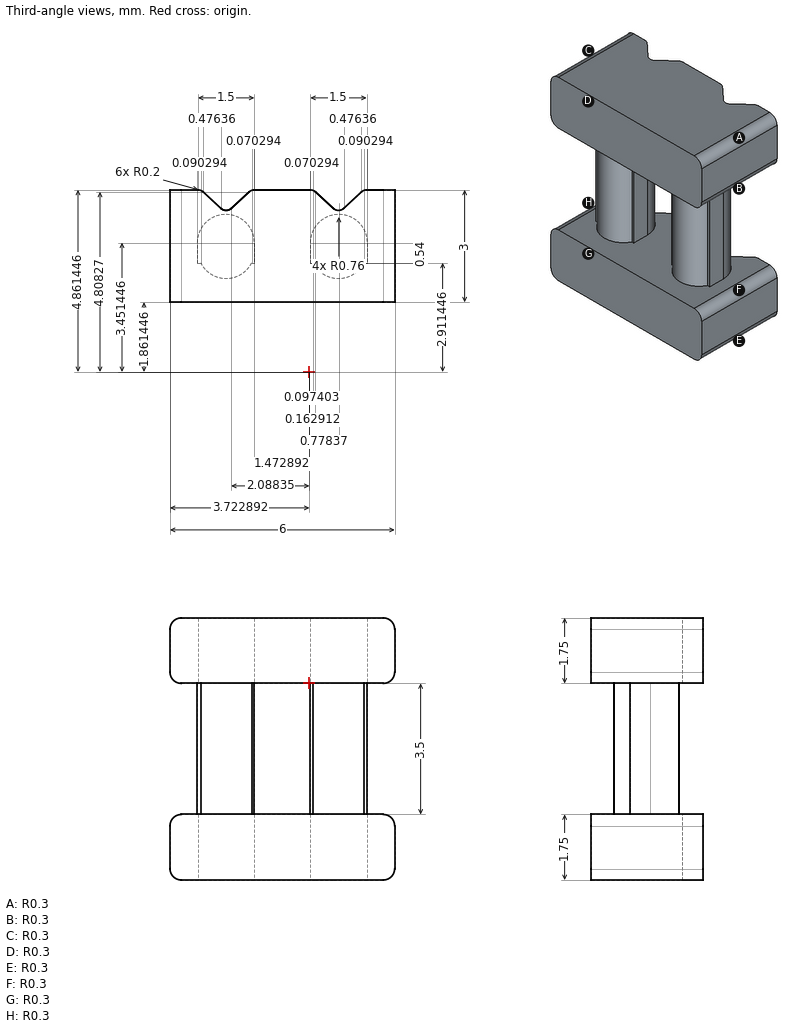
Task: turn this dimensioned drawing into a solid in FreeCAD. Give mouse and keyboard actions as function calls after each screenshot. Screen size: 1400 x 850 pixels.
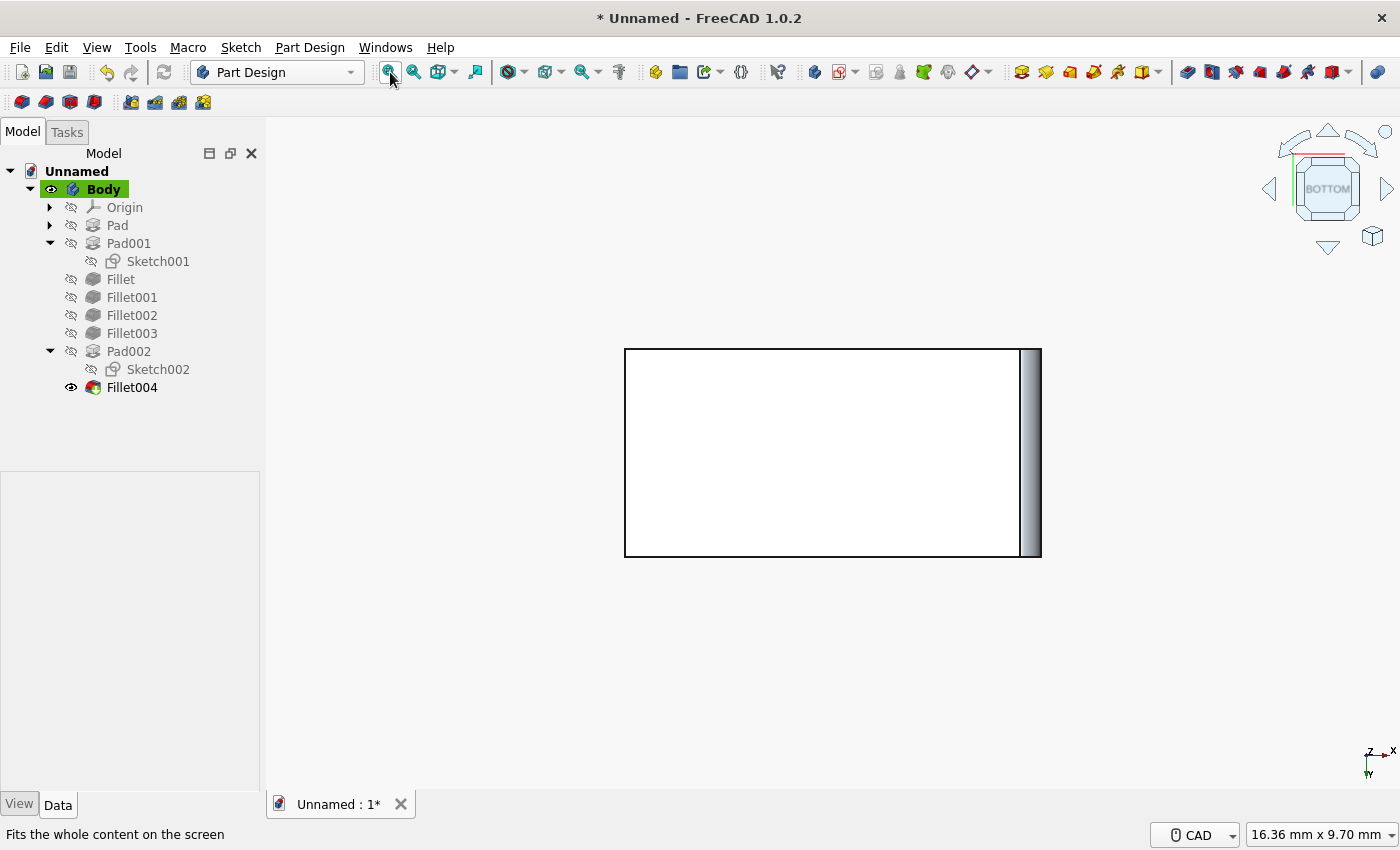
key(0)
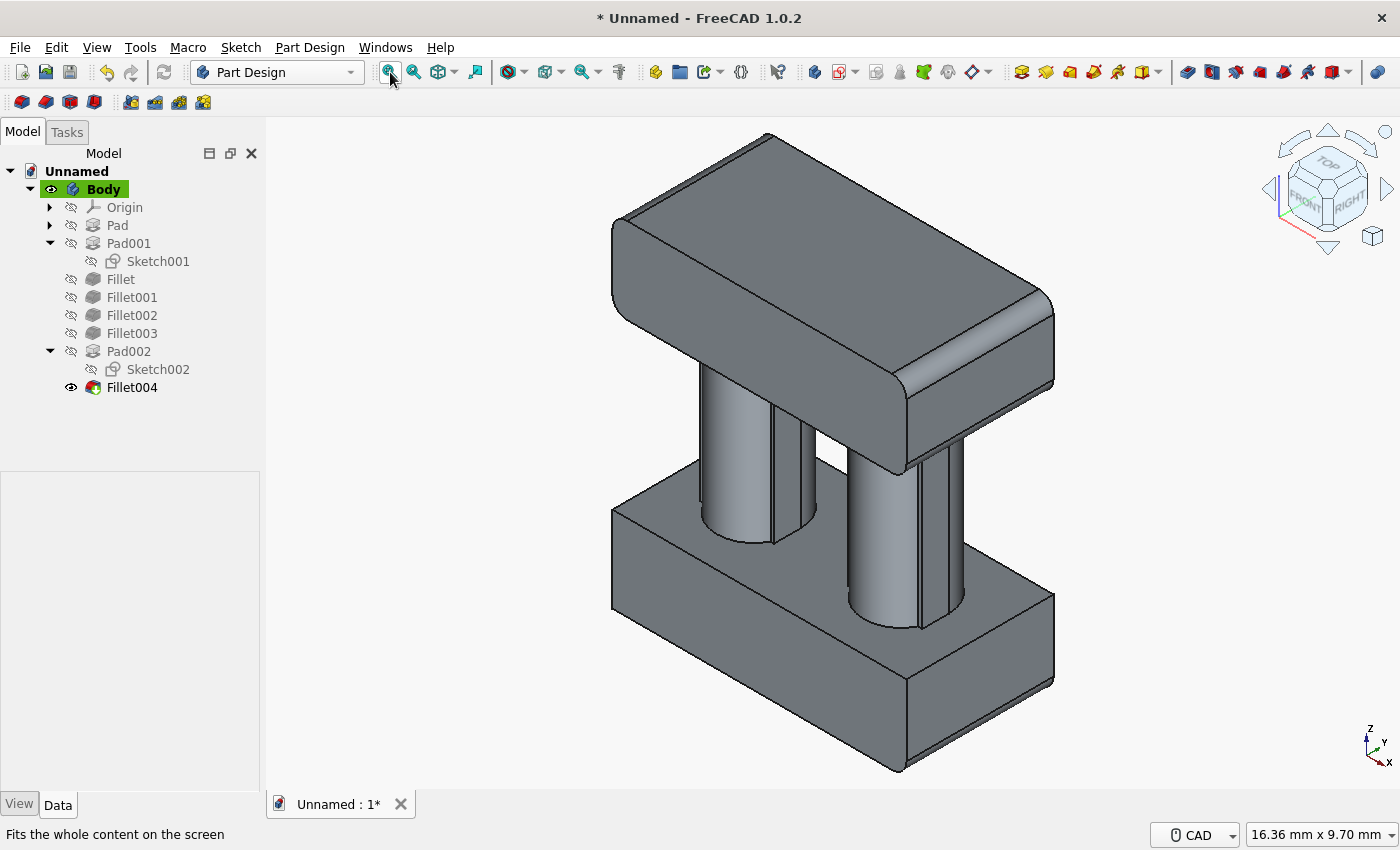
click(980, 636)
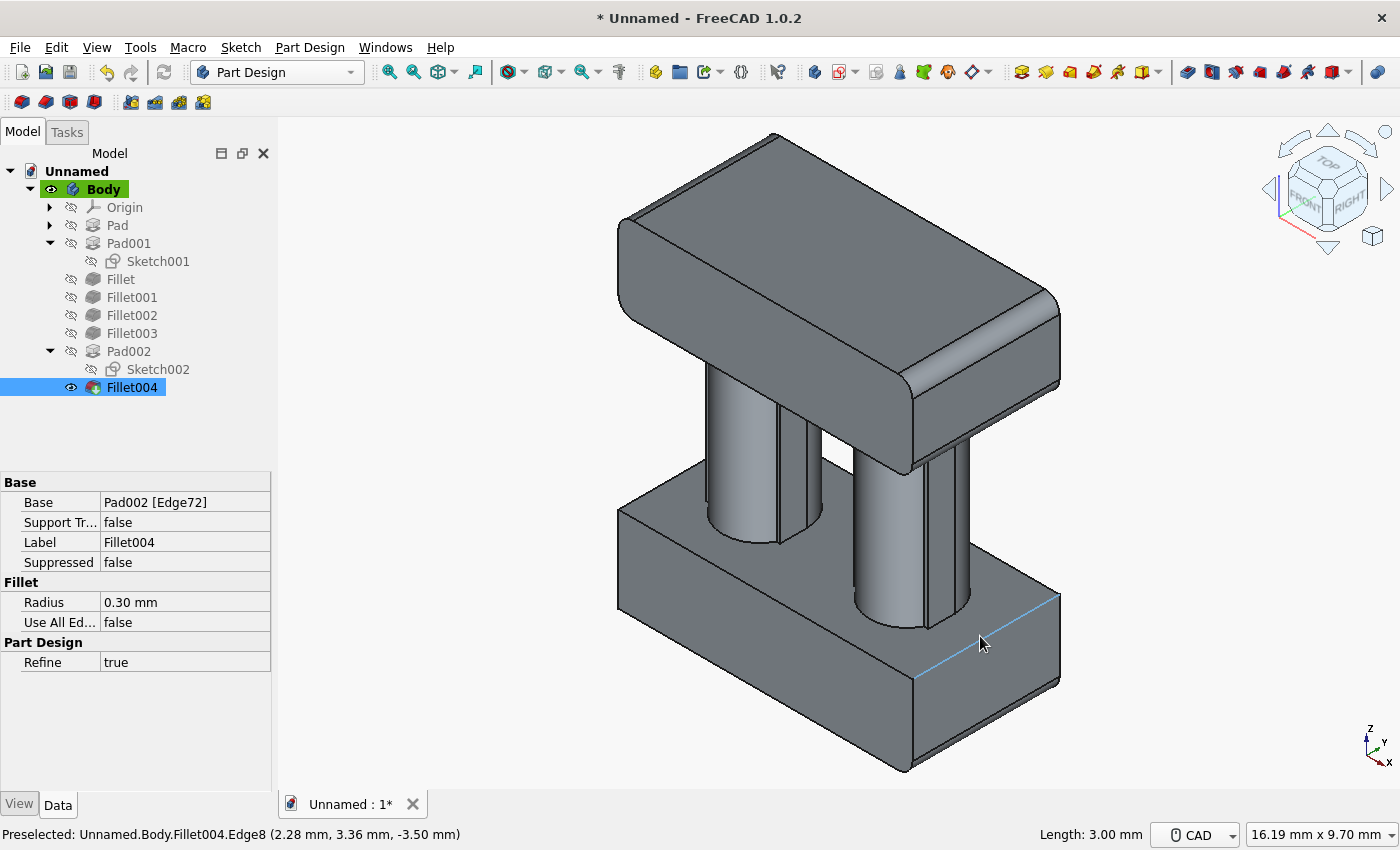
click(22, 102)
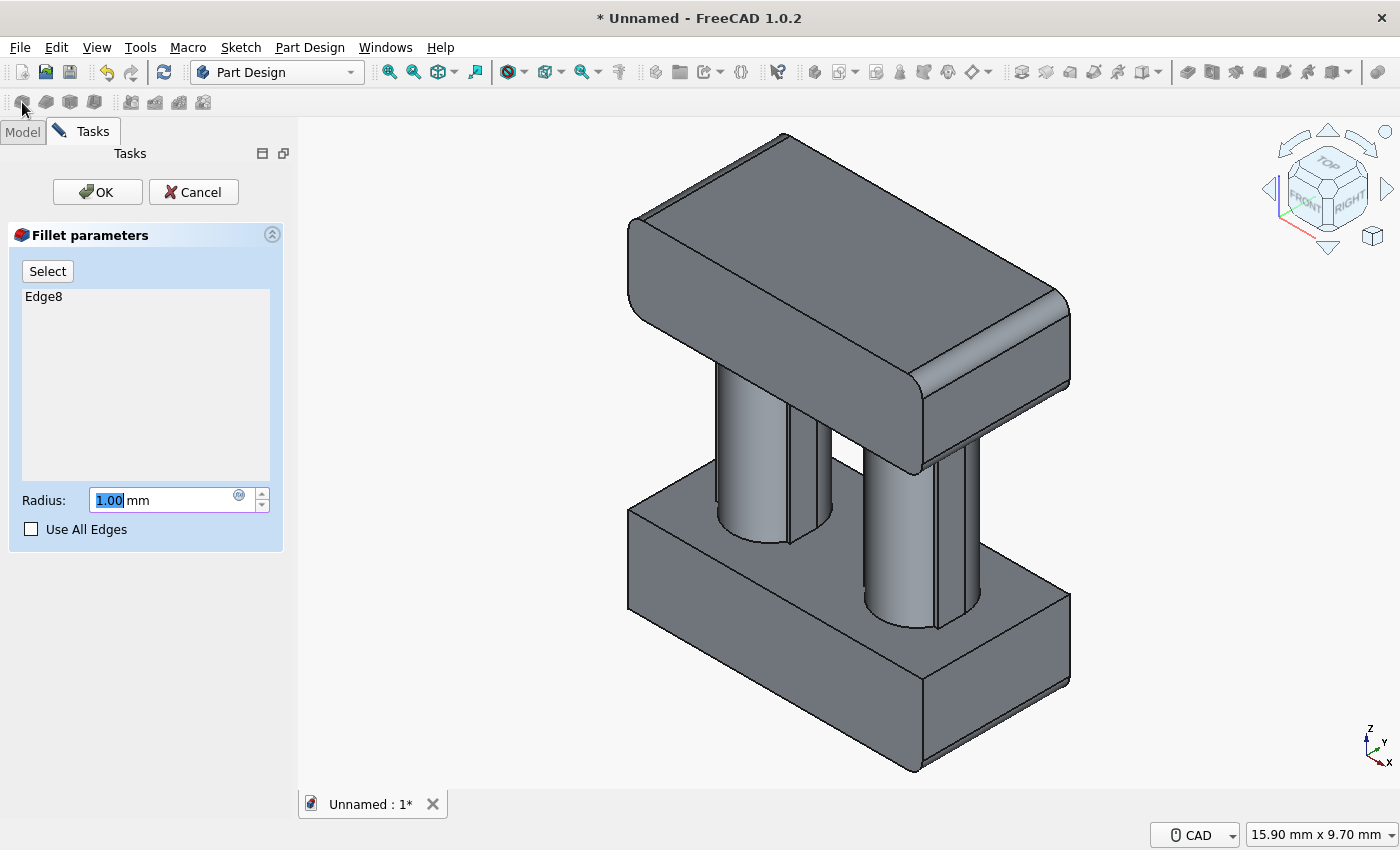
text(0.3)
key(Tab)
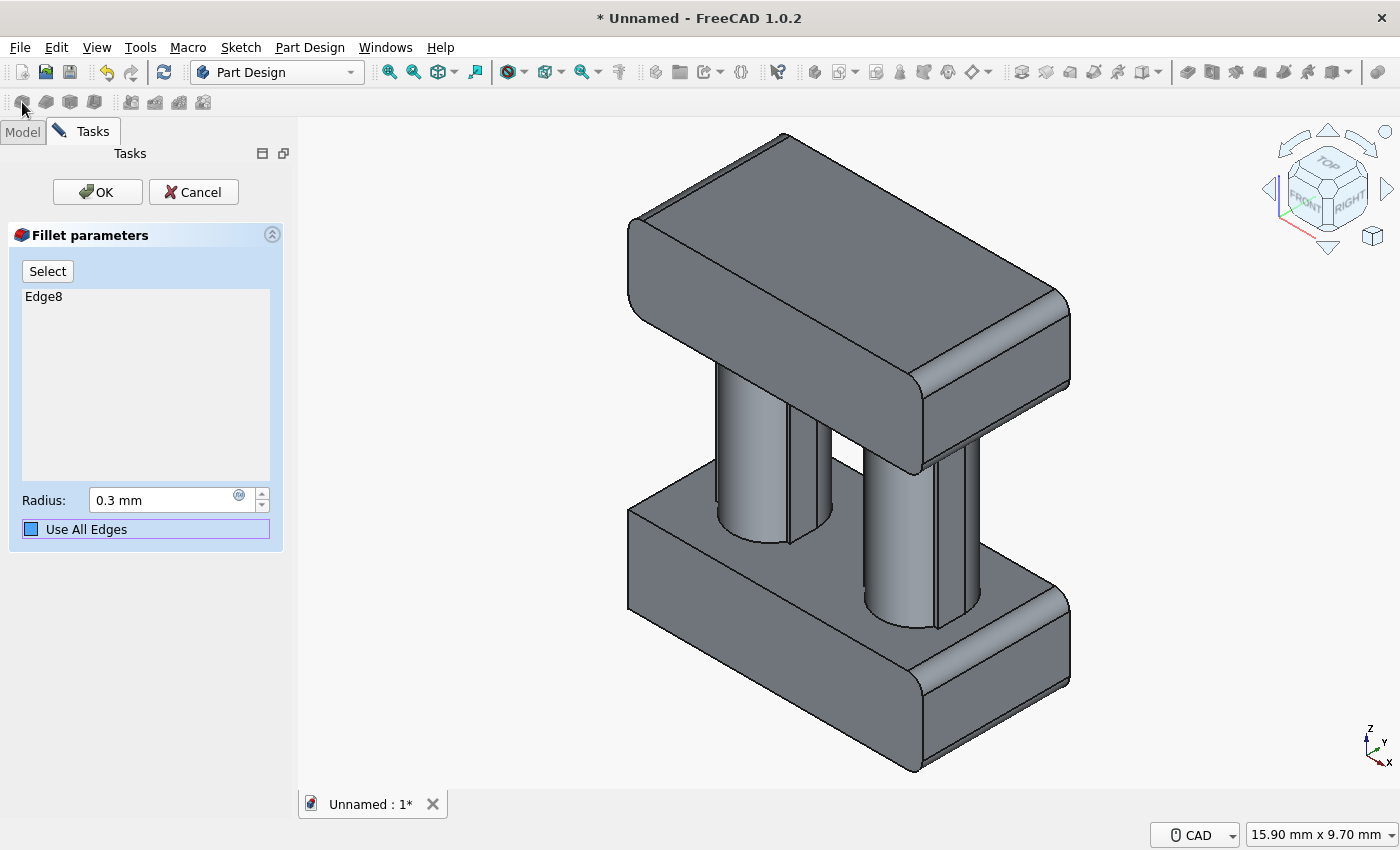
click(98, 192)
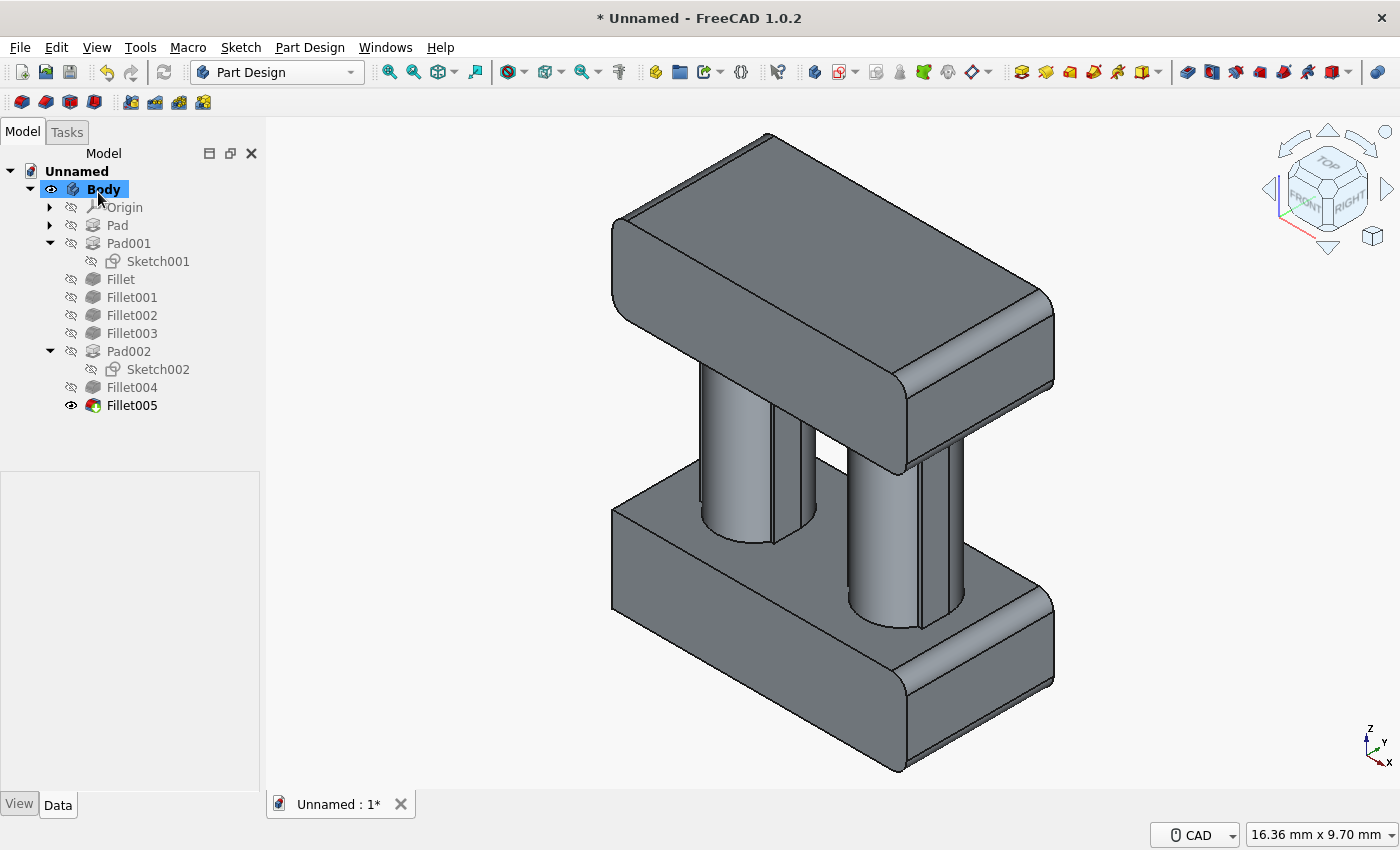
key(2)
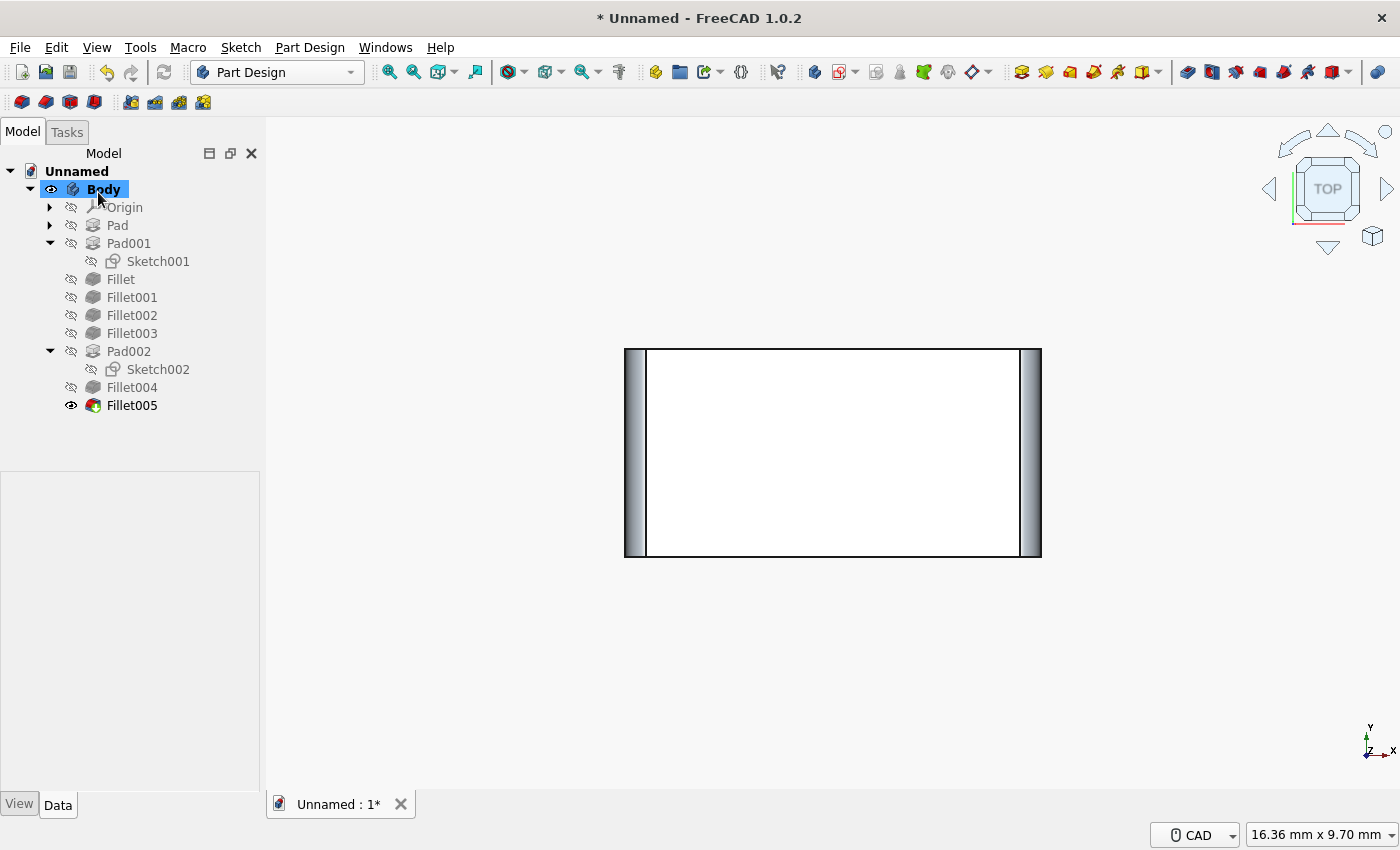
click(390, 72)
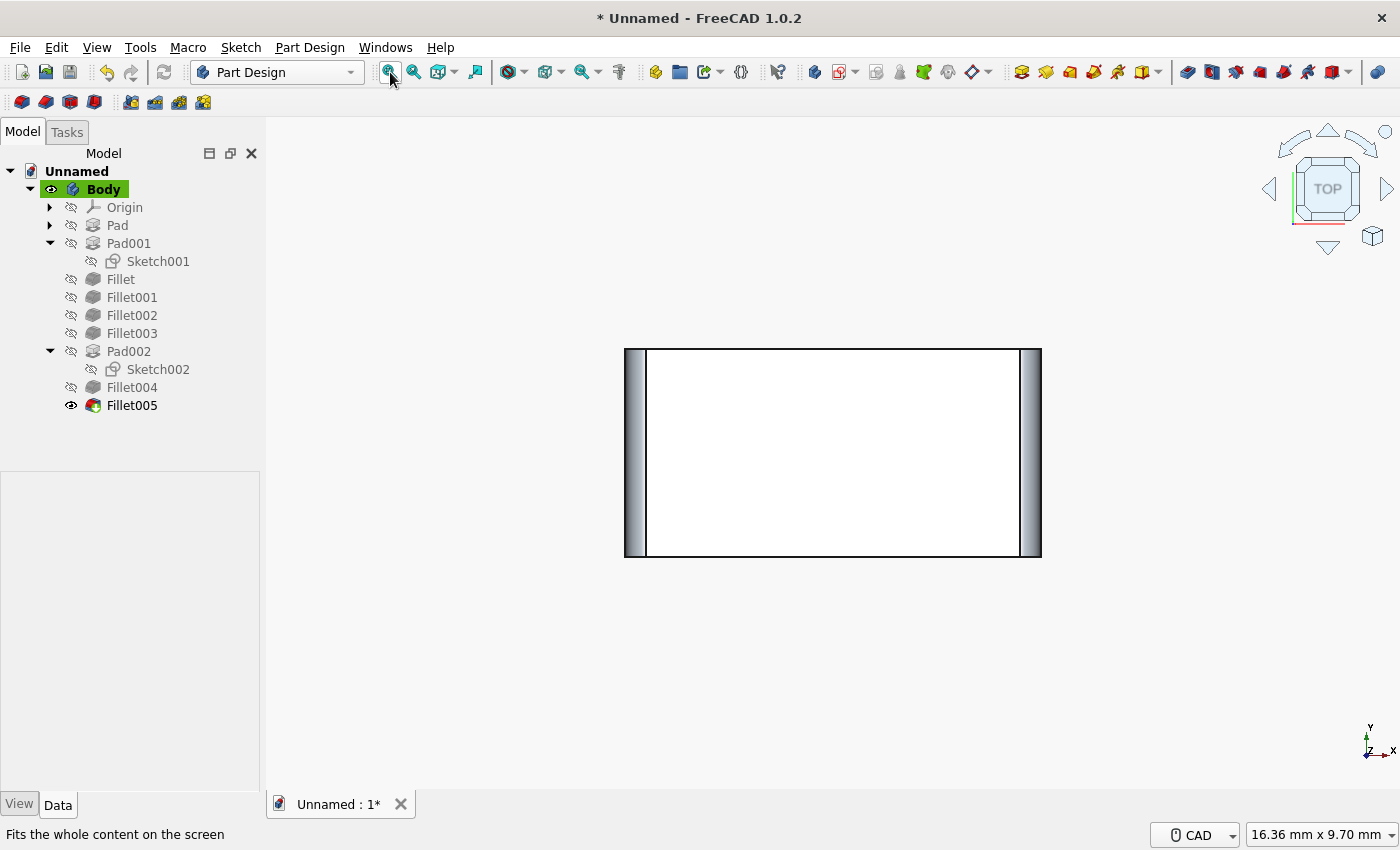
key(0)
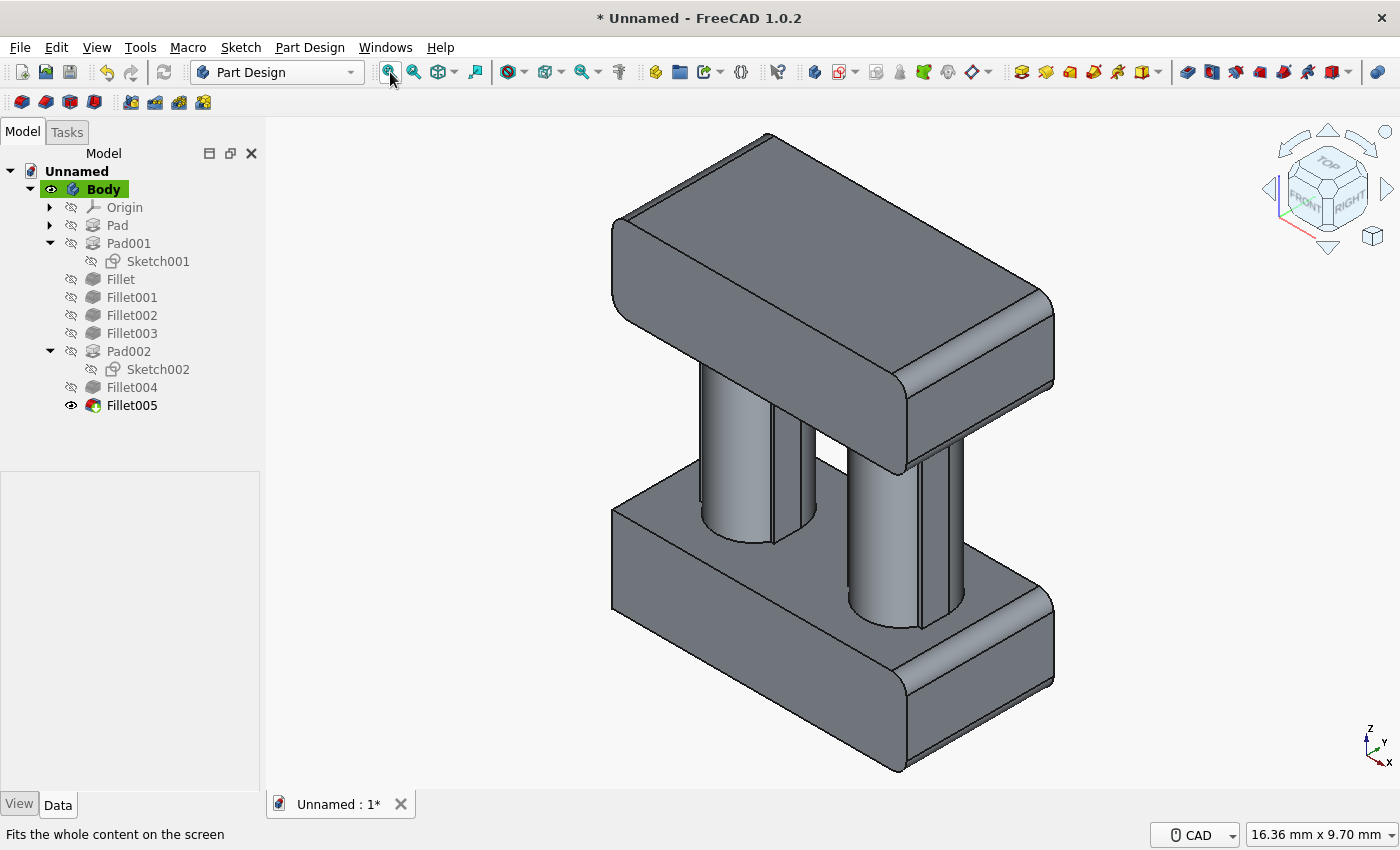
key(1)